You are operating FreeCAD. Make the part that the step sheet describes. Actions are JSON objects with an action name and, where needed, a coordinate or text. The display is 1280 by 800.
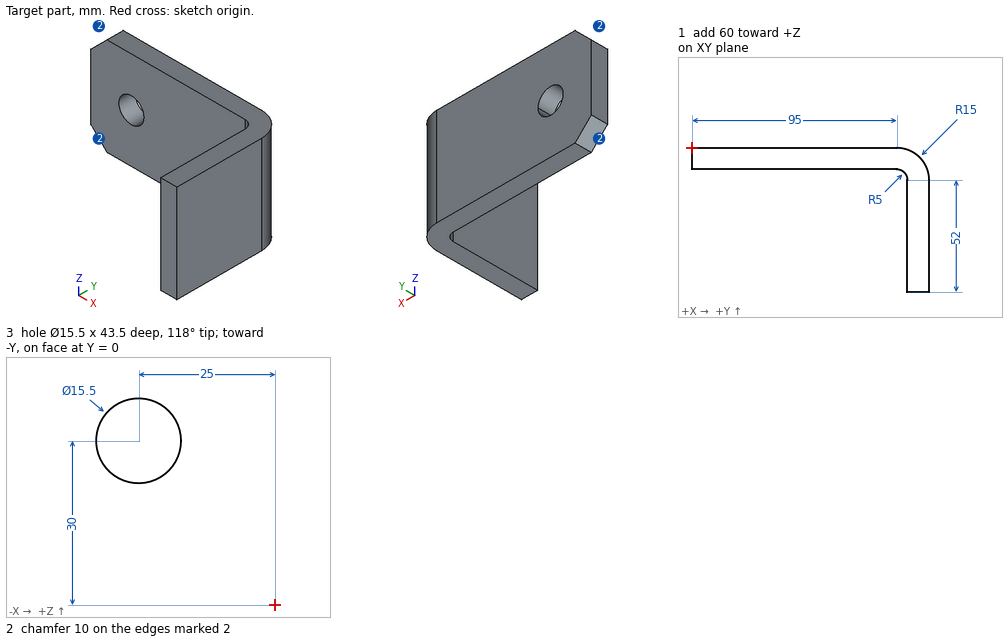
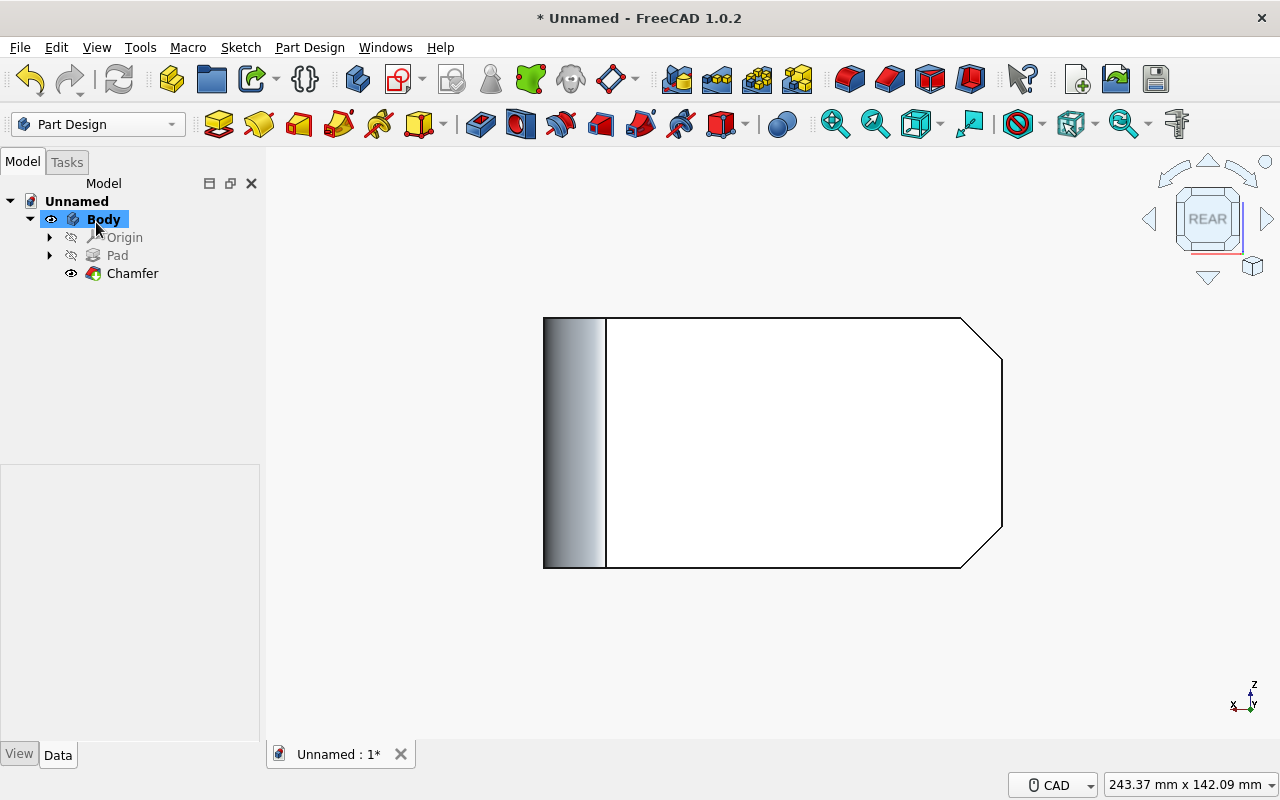
{"action": "left_click", "coordinate": [748, 442]}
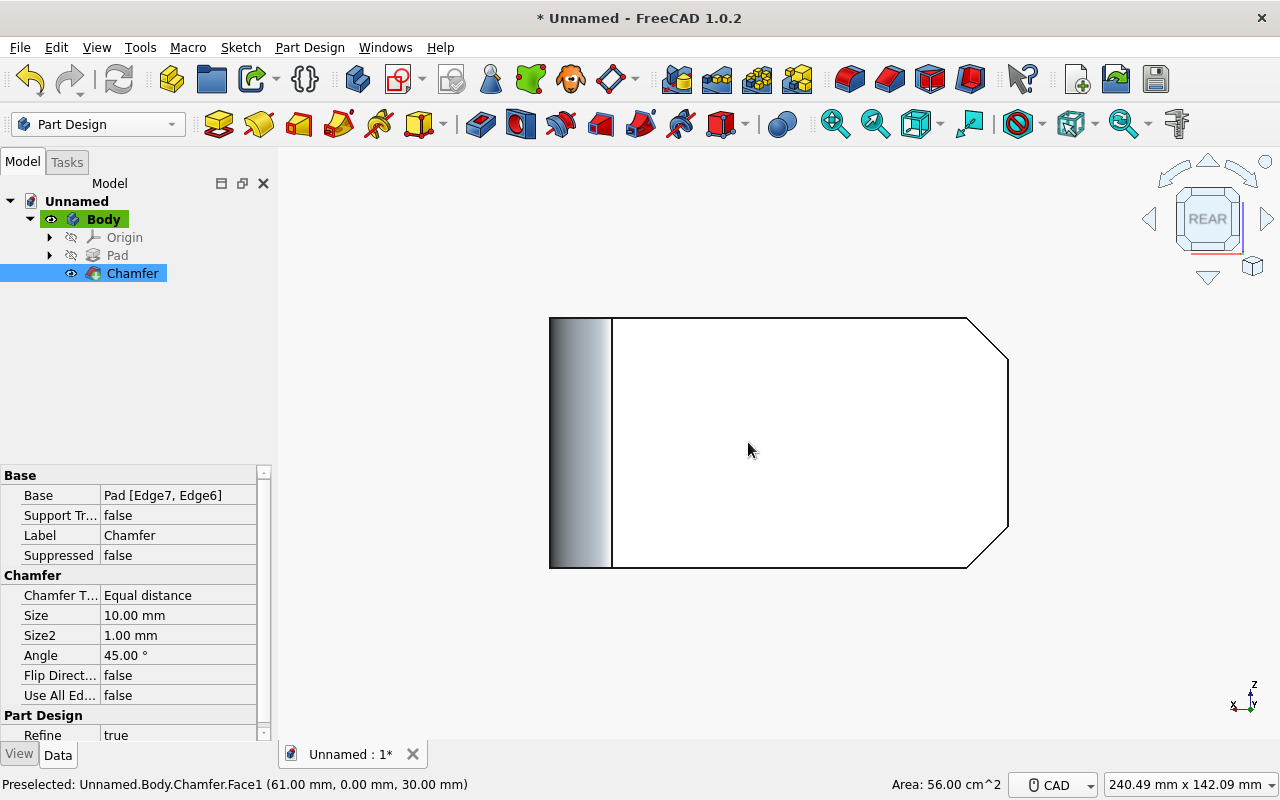
{"action": "left_click", "coordinate": [398, 80]}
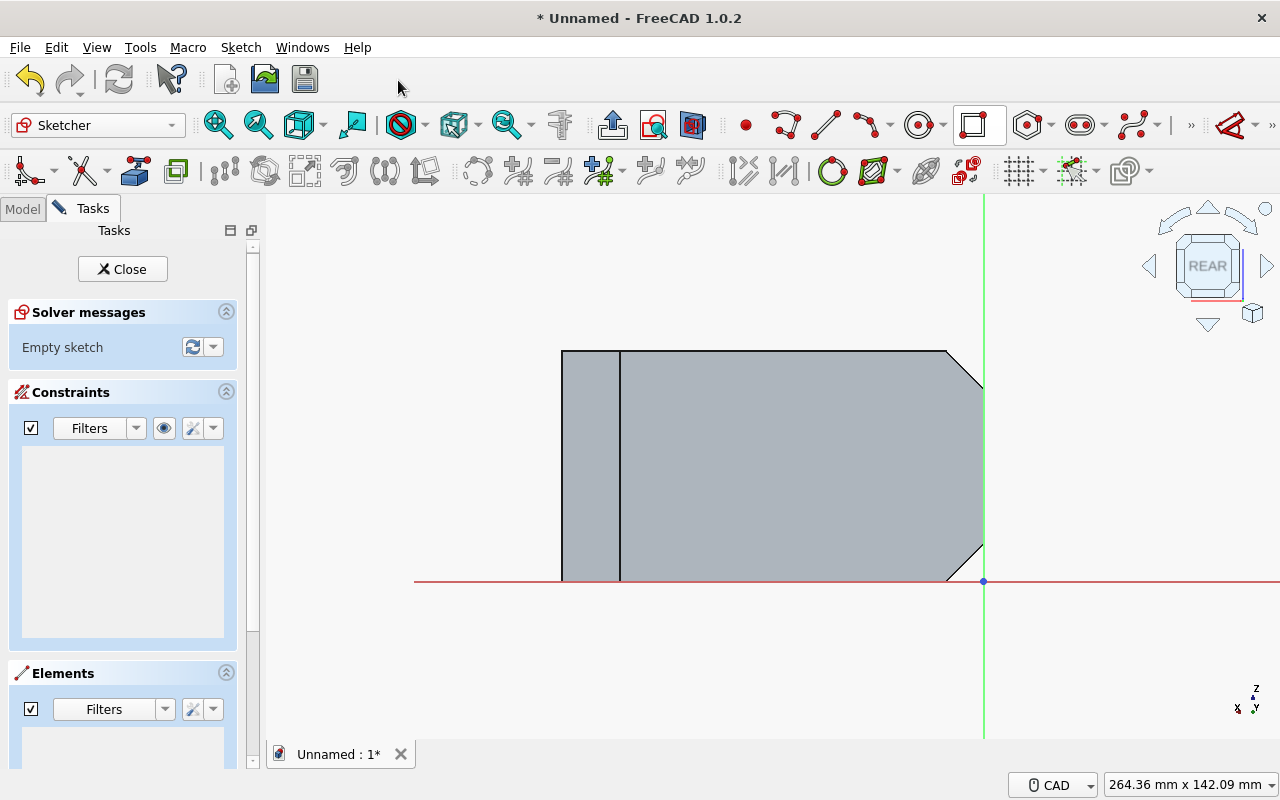
{"action": "scroll", "coordinate": [1098, 544], "scroll_direction": "up", "scroll_amount": 4}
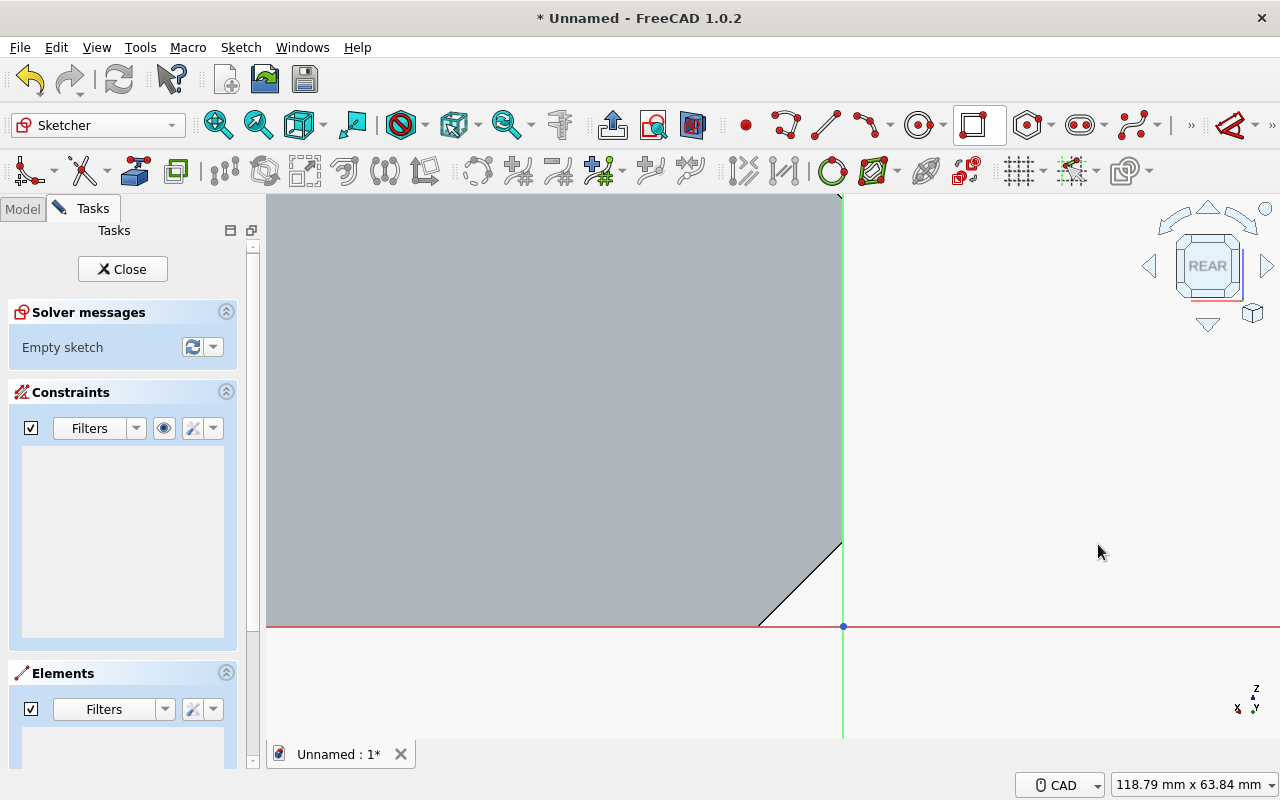
{"action": "key", "text": "g c"}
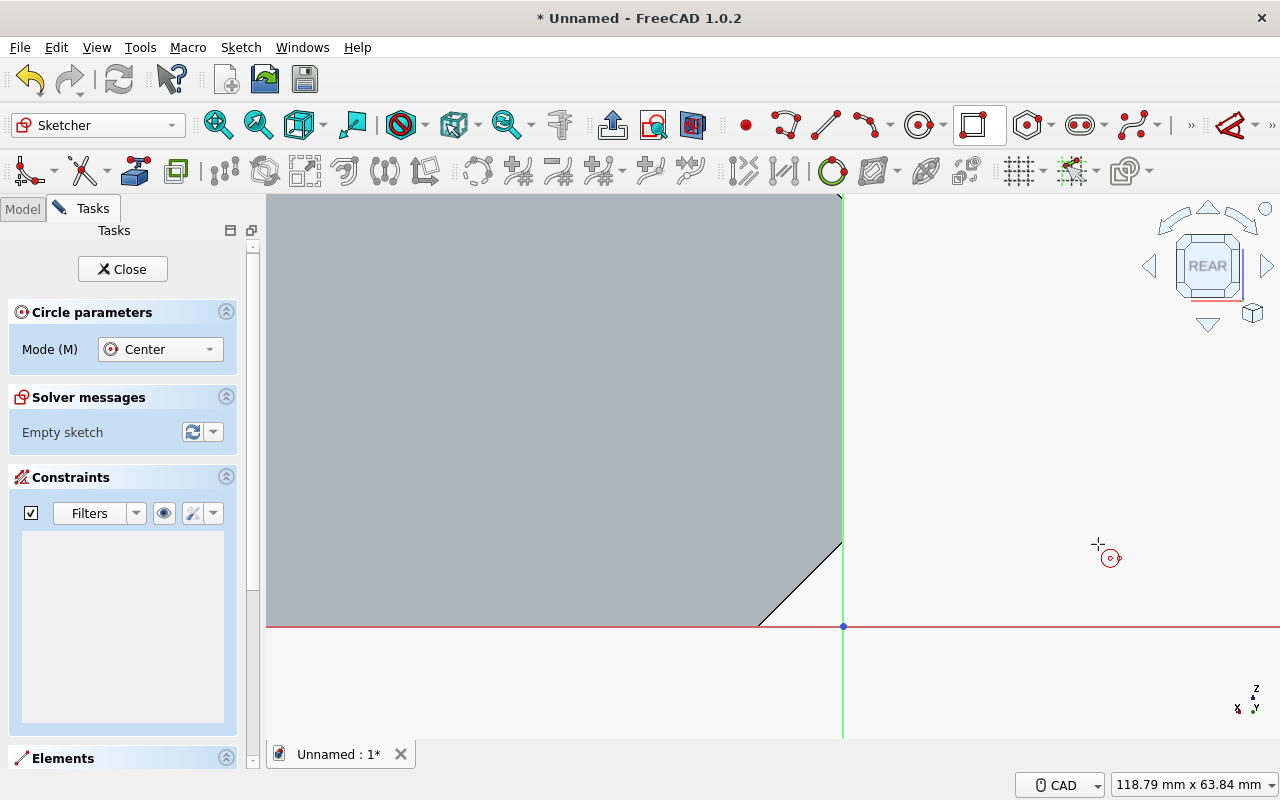
{"action": "left_click", "coordinate": [630, 371]}
{"action": "mouse_move", "coordinate": [677, 324]}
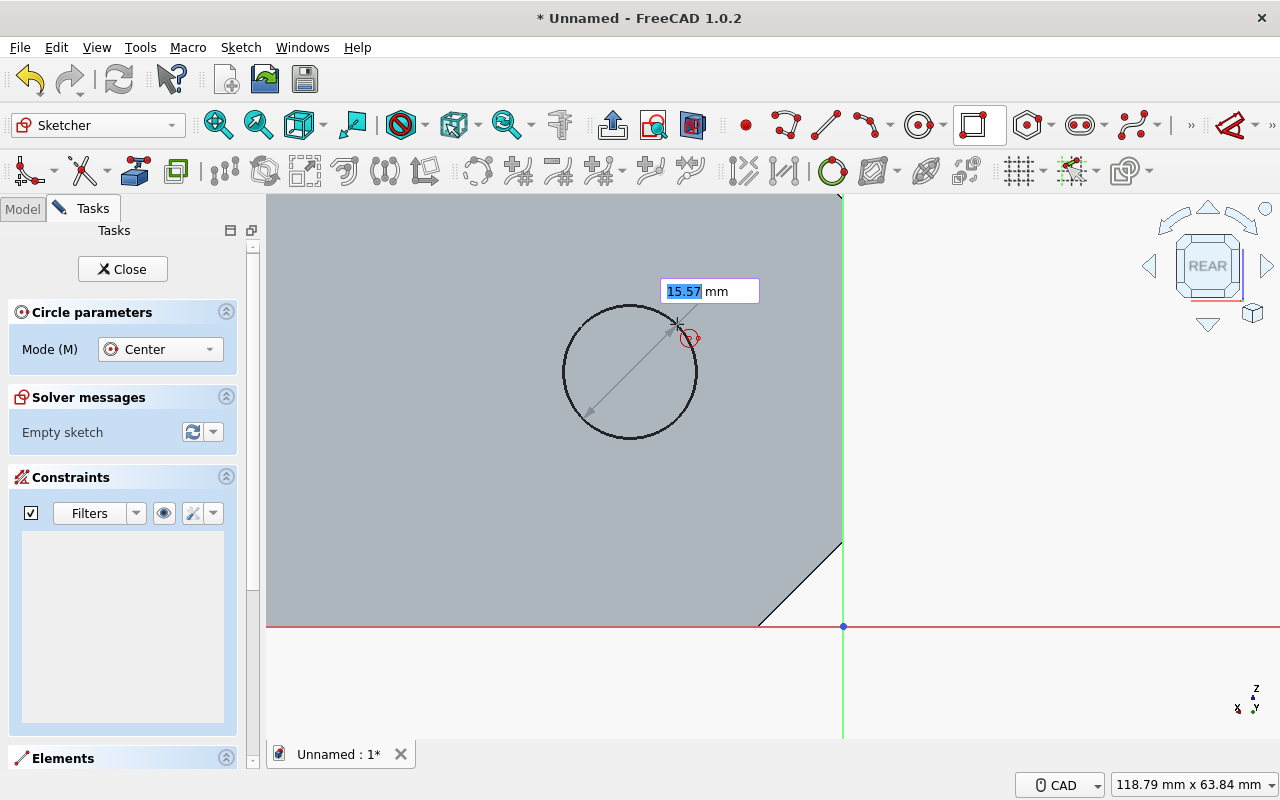
{"action": "type", "text": "15.5"}
{"action": "key", "text": "Return"}
{"action": "key", "text": "Escape"}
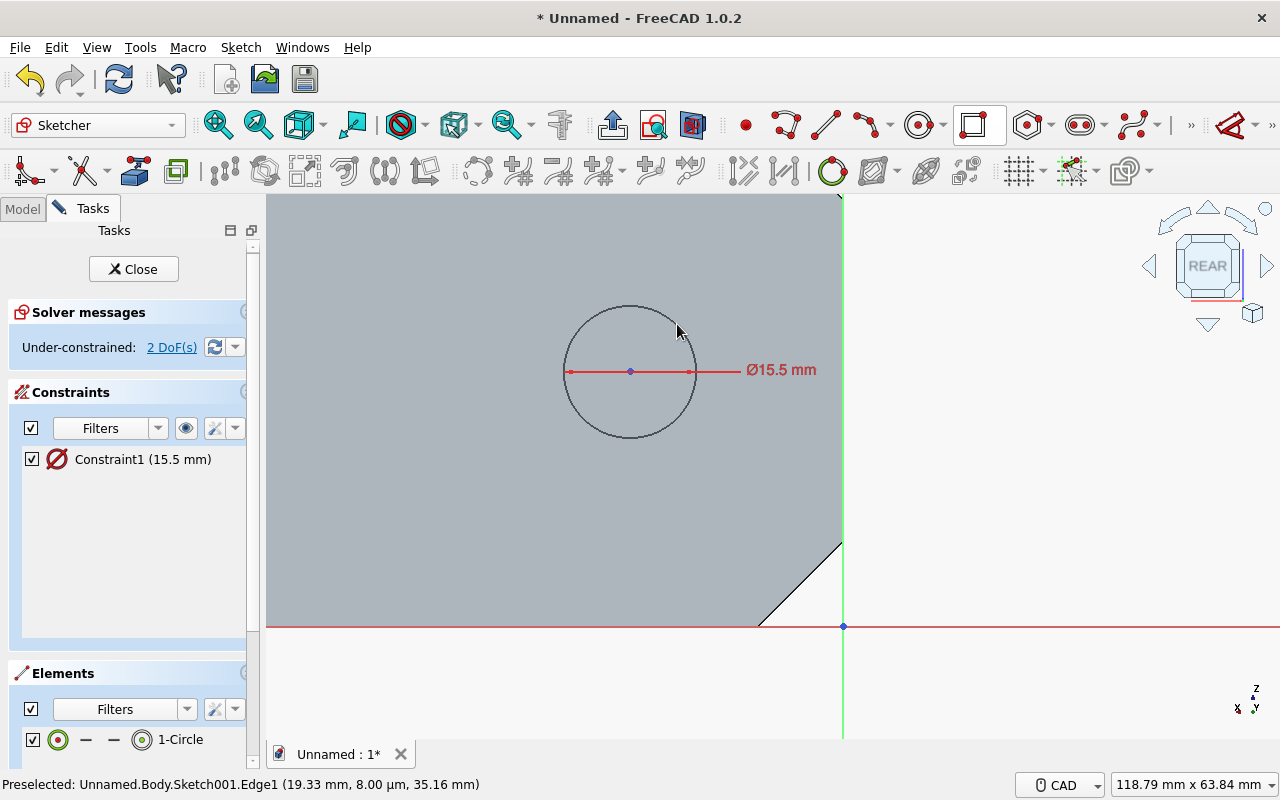
{"action": "left_click", "coordinate": [1230, 126]}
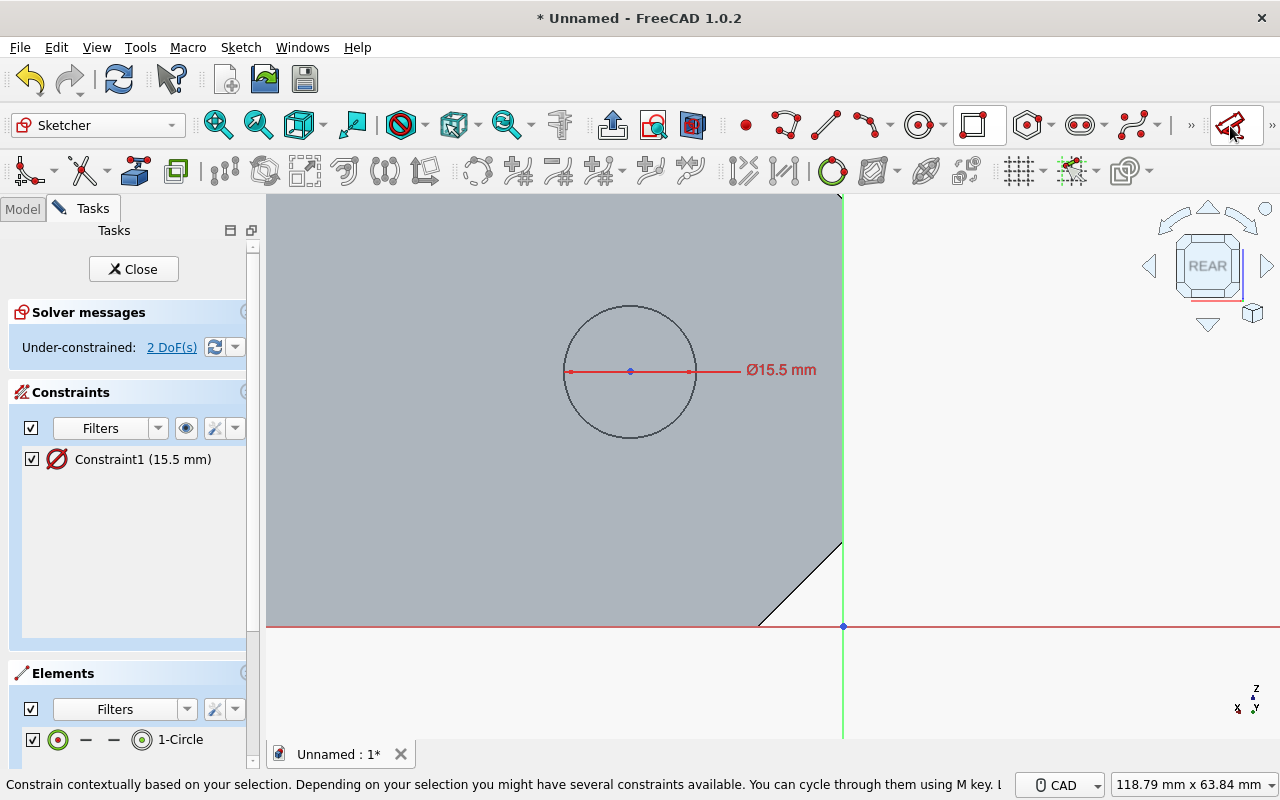
{"action": "left_click", "coordinate": [630, 372]}
{"action": "left_click", "coordinate": [737, 661]}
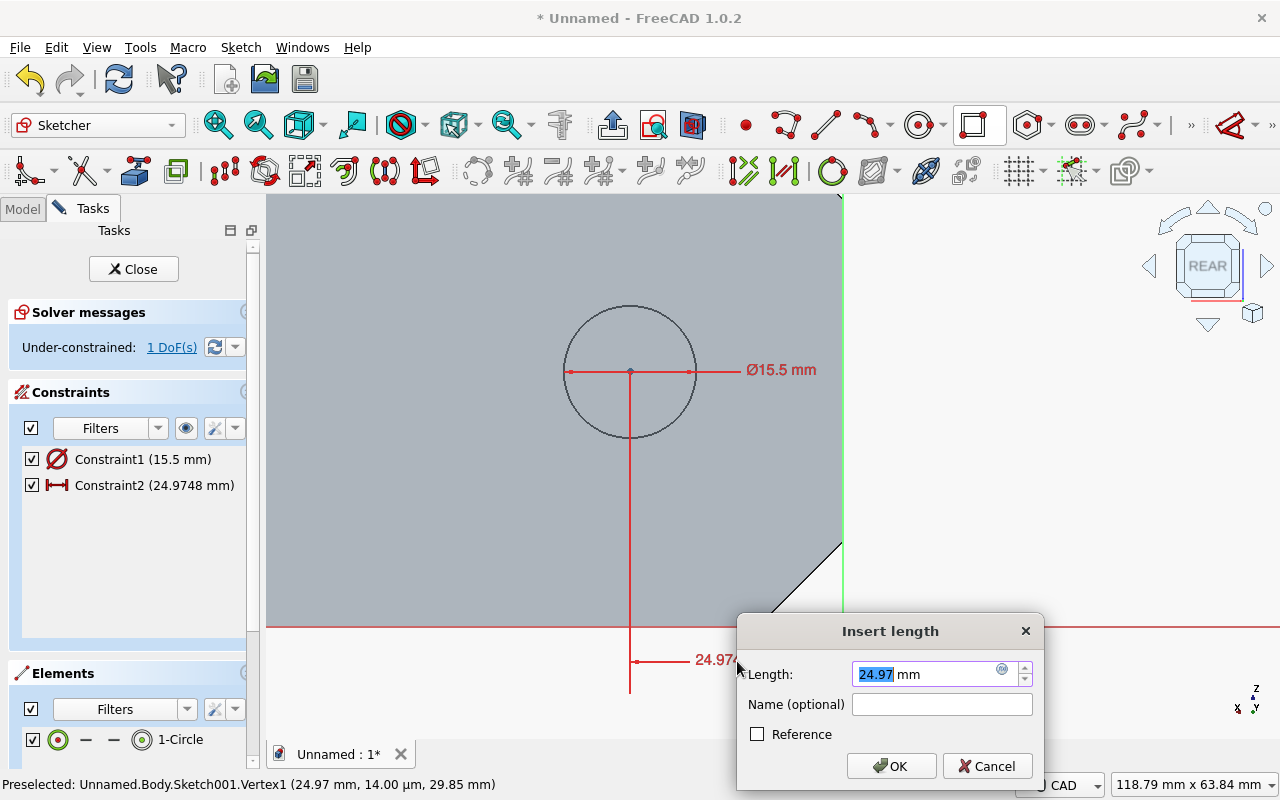
{"action": "type", "text": "25"}
{"action": "key", "text": "Return"}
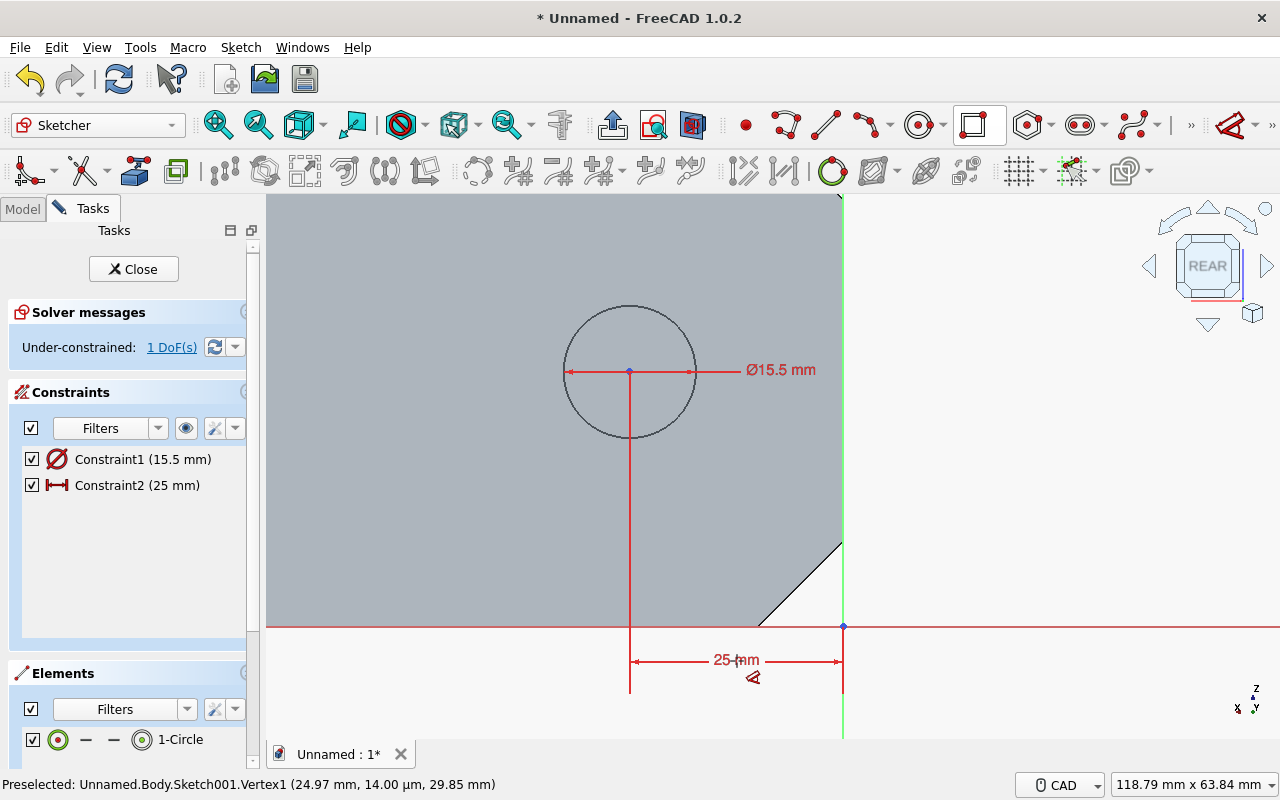
{"action": "left_click", "coordinate": [630, 372]}
{"action": "left_click", "coordinate": [877, 499]}